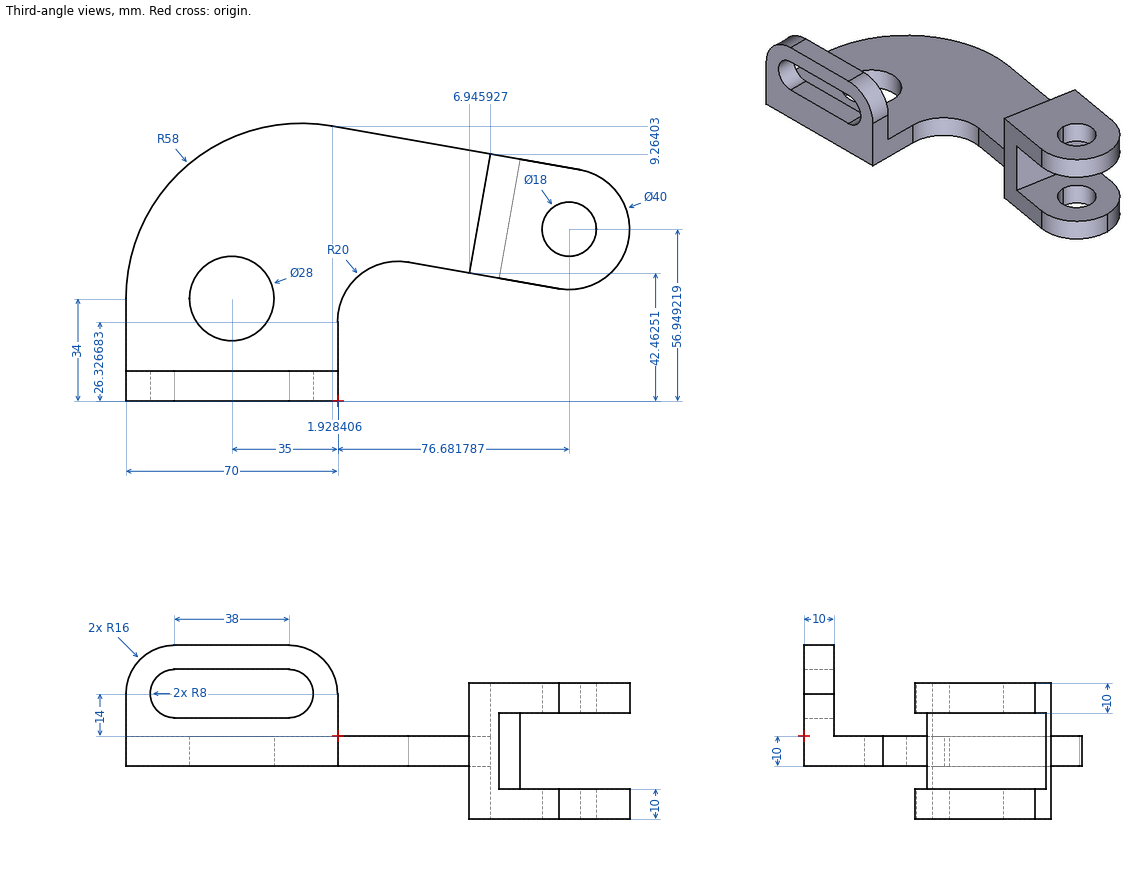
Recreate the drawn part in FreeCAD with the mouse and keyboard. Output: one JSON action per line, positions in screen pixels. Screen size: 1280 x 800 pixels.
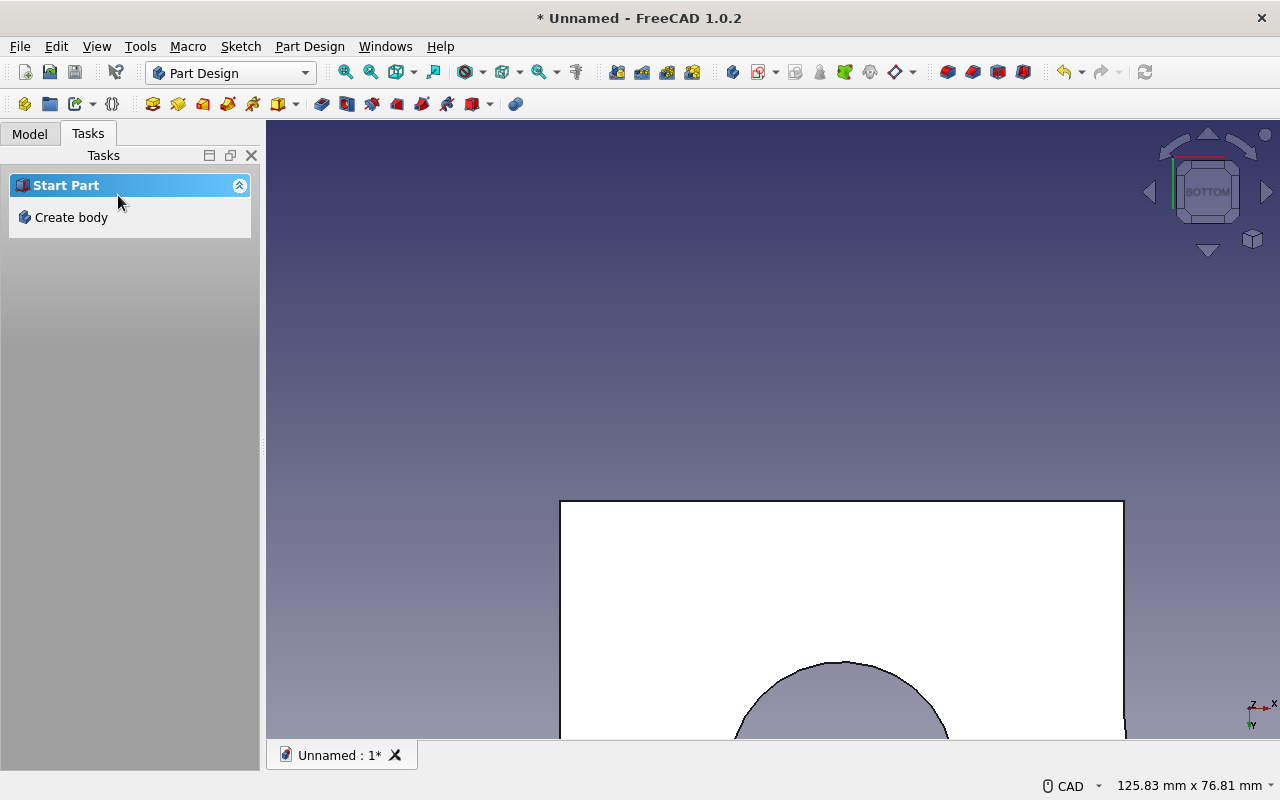
{"action": "left_click", "coordinate": [346, 72]}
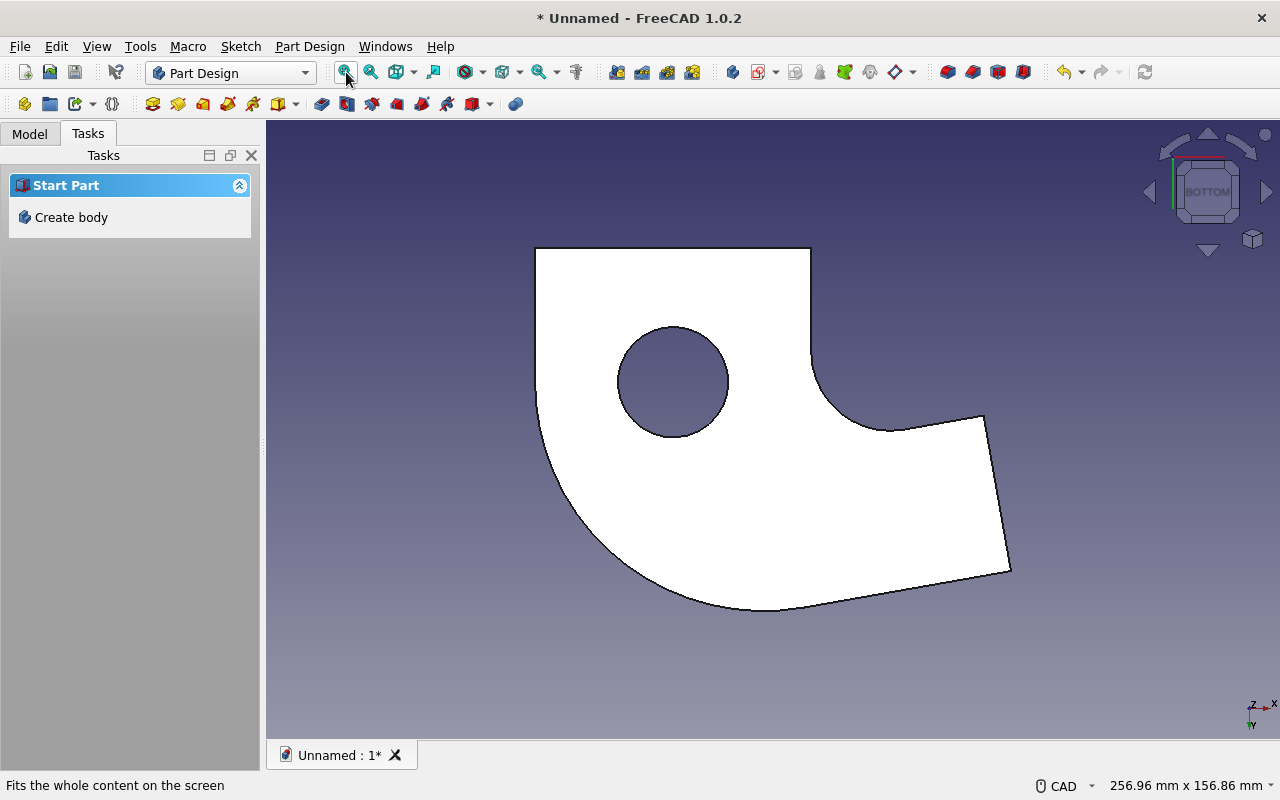
{"action": "key", "text": "4"}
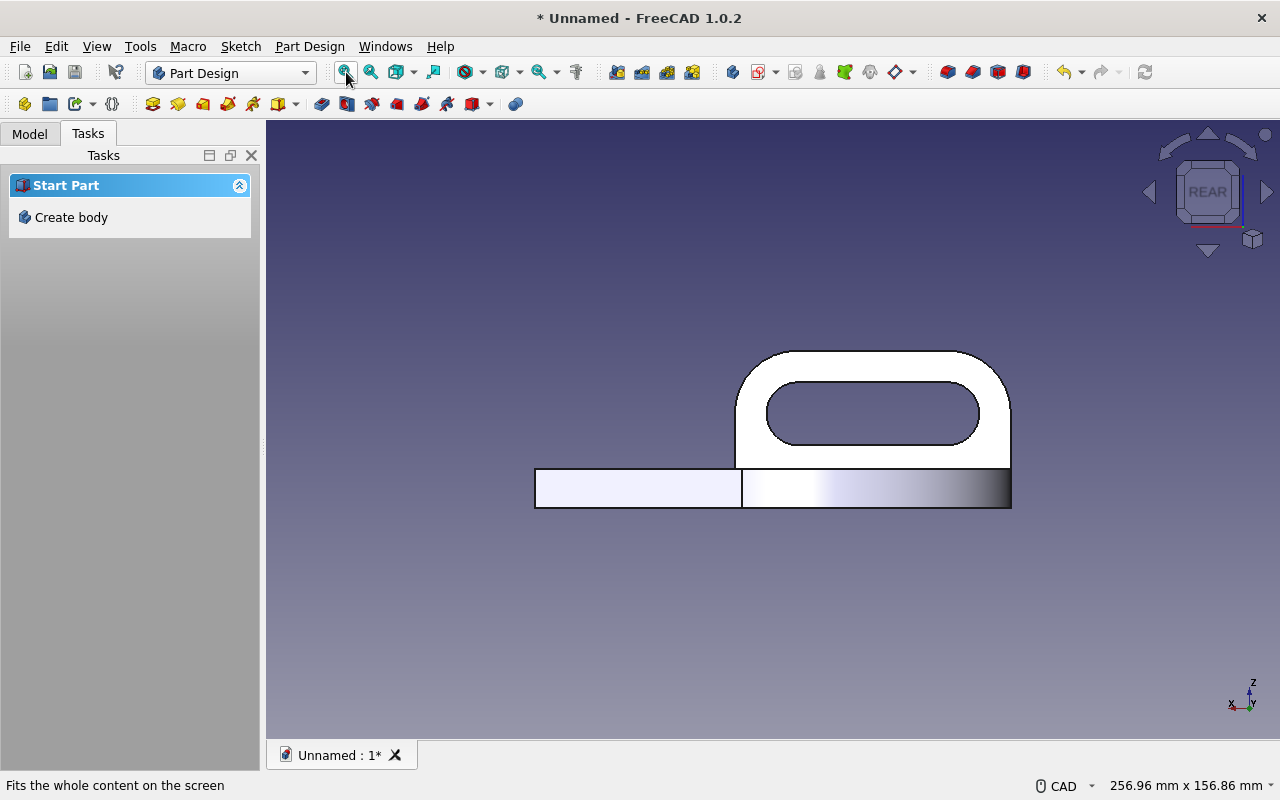
{"action": "left_click", "coordinate": [579, 488]}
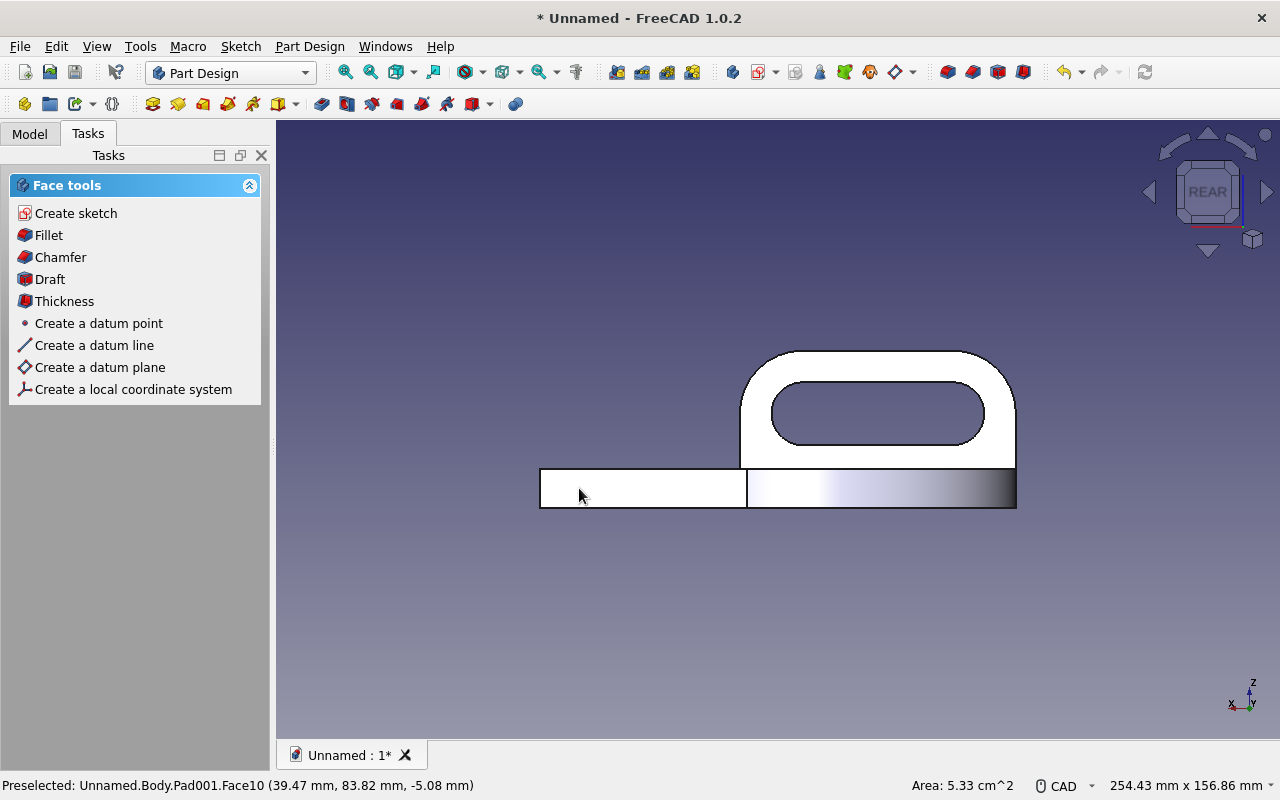
{"action": "left_click", "coordinate": [758, 72]}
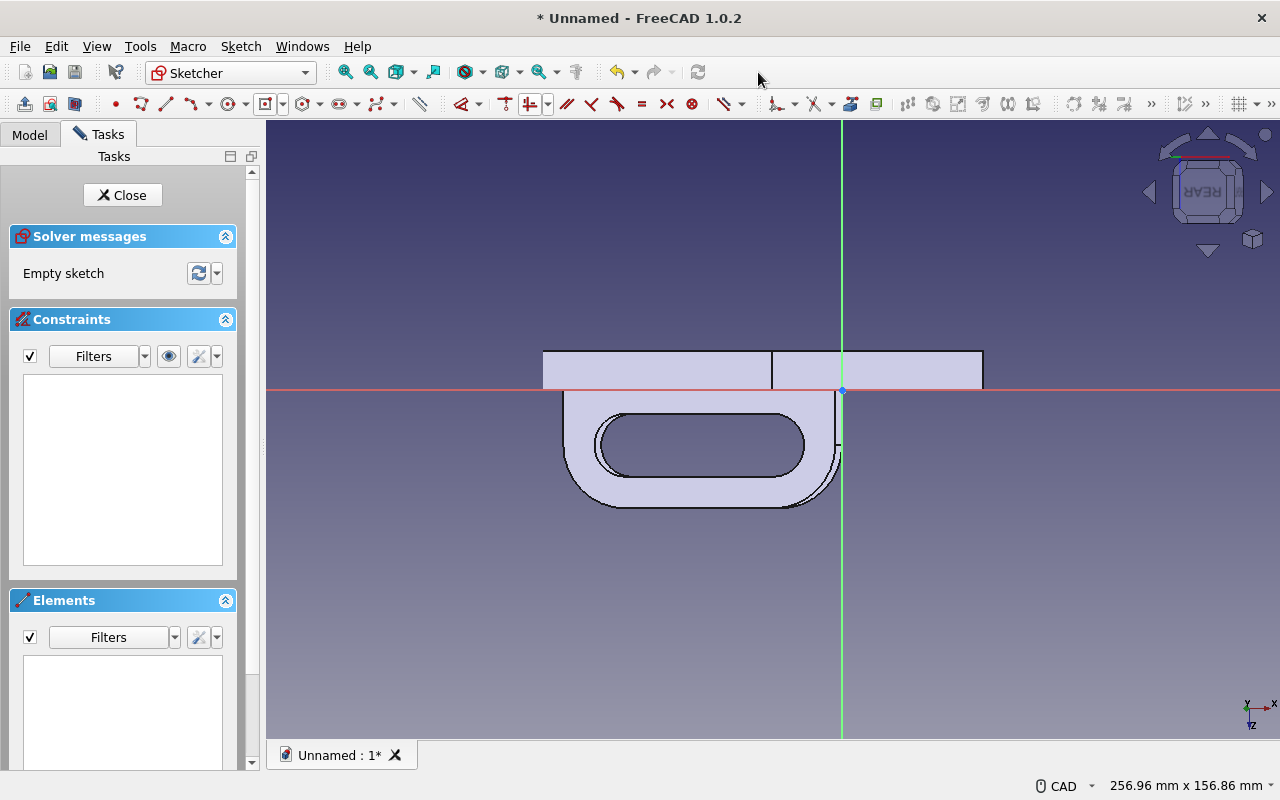
{"action": "left_click", "coordinate": [75, 104]}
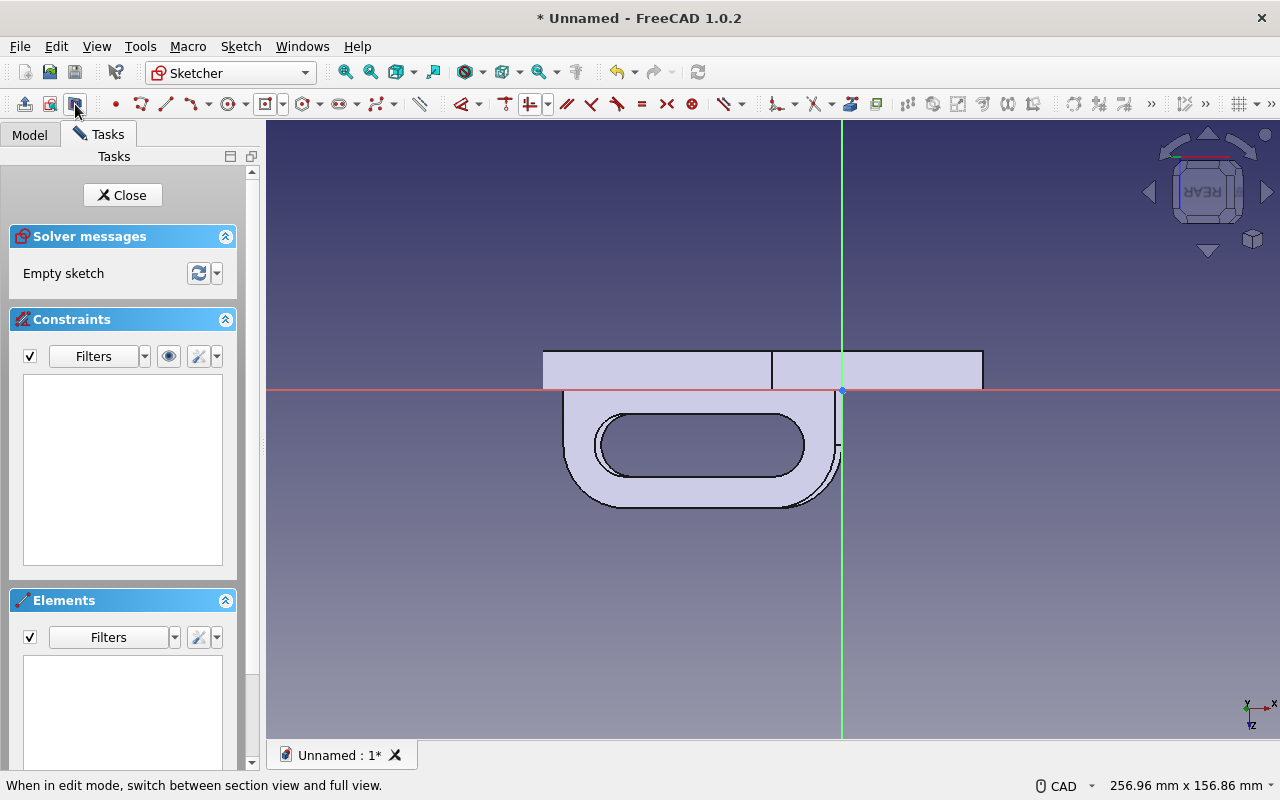
{"action": "scroll", "coordinate": [1115, 322], "scroll_direction": "up", "scroll_amount": 4}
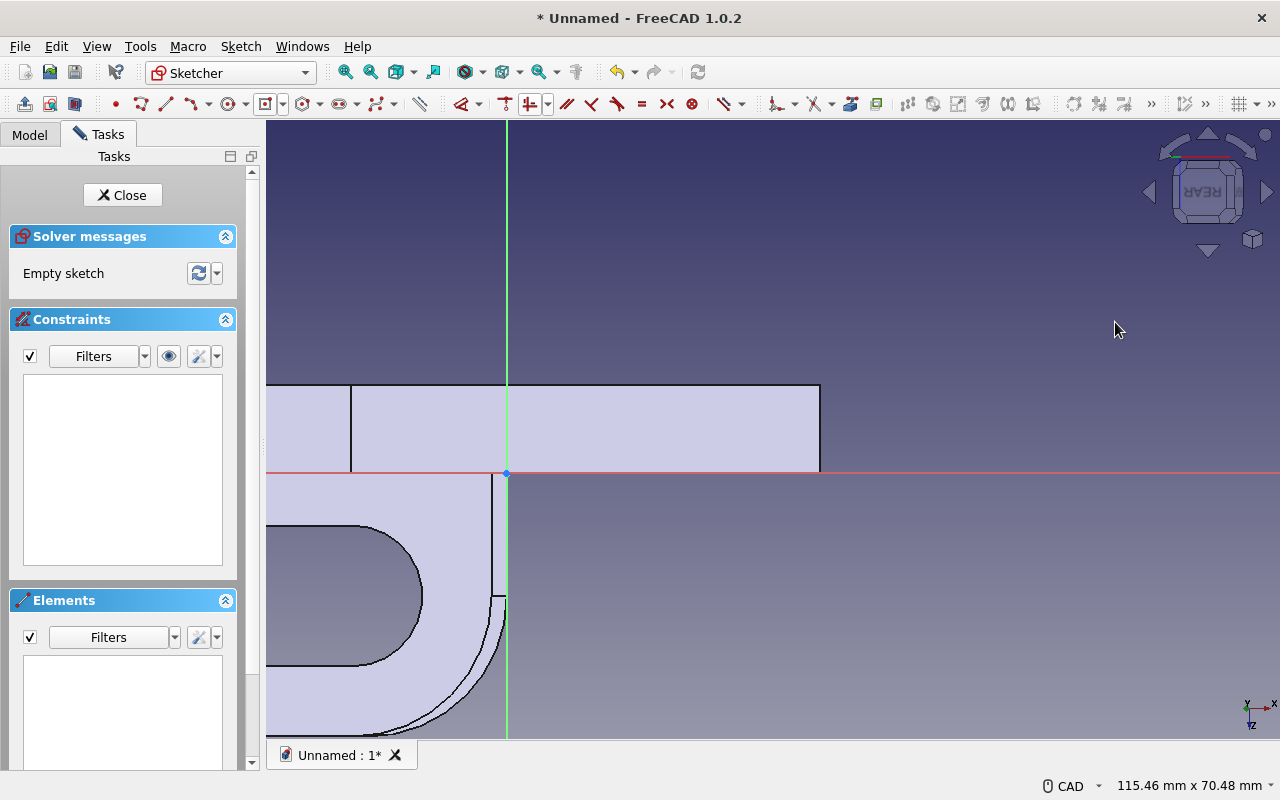
{"action": "left_click", "coordinate": [141, 104]}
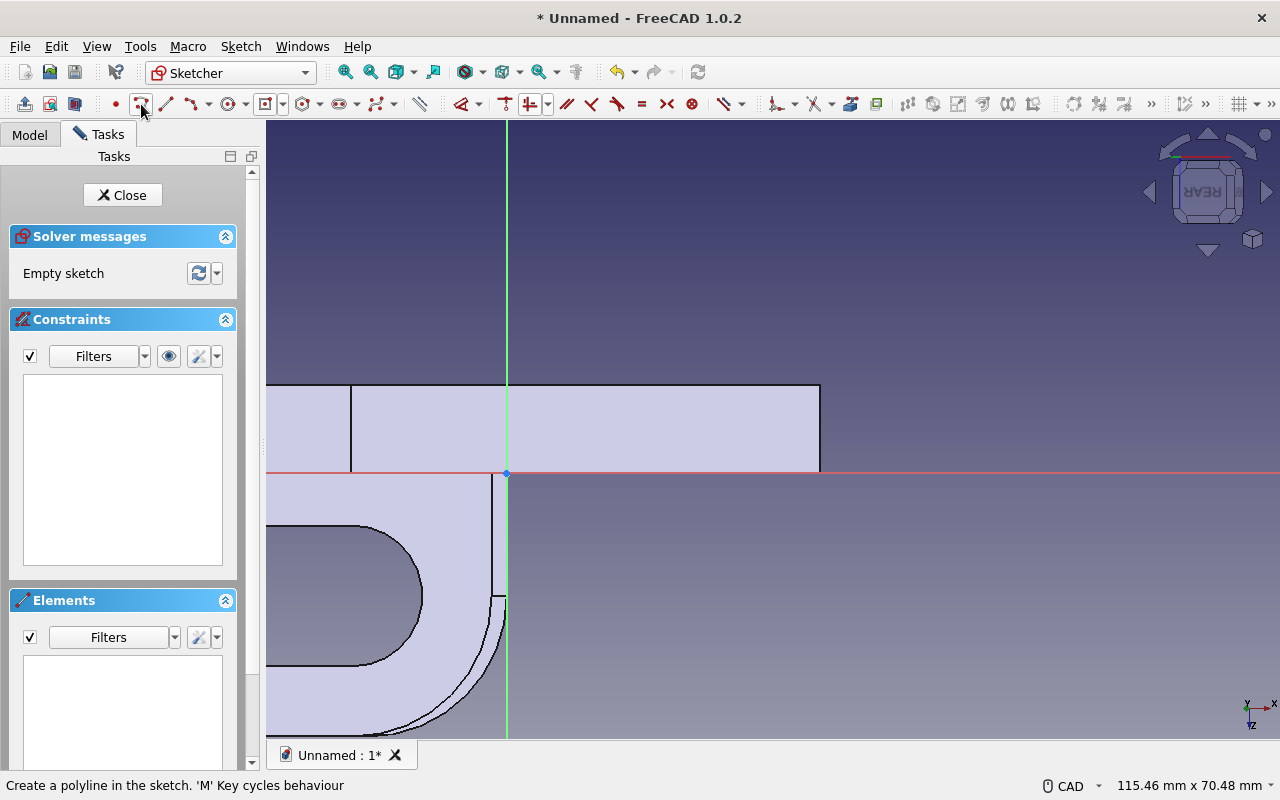
{"action": "left_click", "coordinate": [820, 627]}
{"action": "left_click", "coordinate": [1083, 627]}
{"action": "left_click", "coordinate": [1083, 539]}
{"action": "left_click", "coordinate": [908, 539]}
{"action": "left_click", "coordinate": [908, 319]}
{"action": "left_click", "coordinate": [1083, 319]}
{"action": "left_click", "coordinate": [1083, 232]}
{"action": "left_click", "coordinate": [820, 232]}
{"action": "left_click", "coordinate": [820, 628]}
{"action": "key", "text": "Escape"}
{"action": "key", "text": "Escape"}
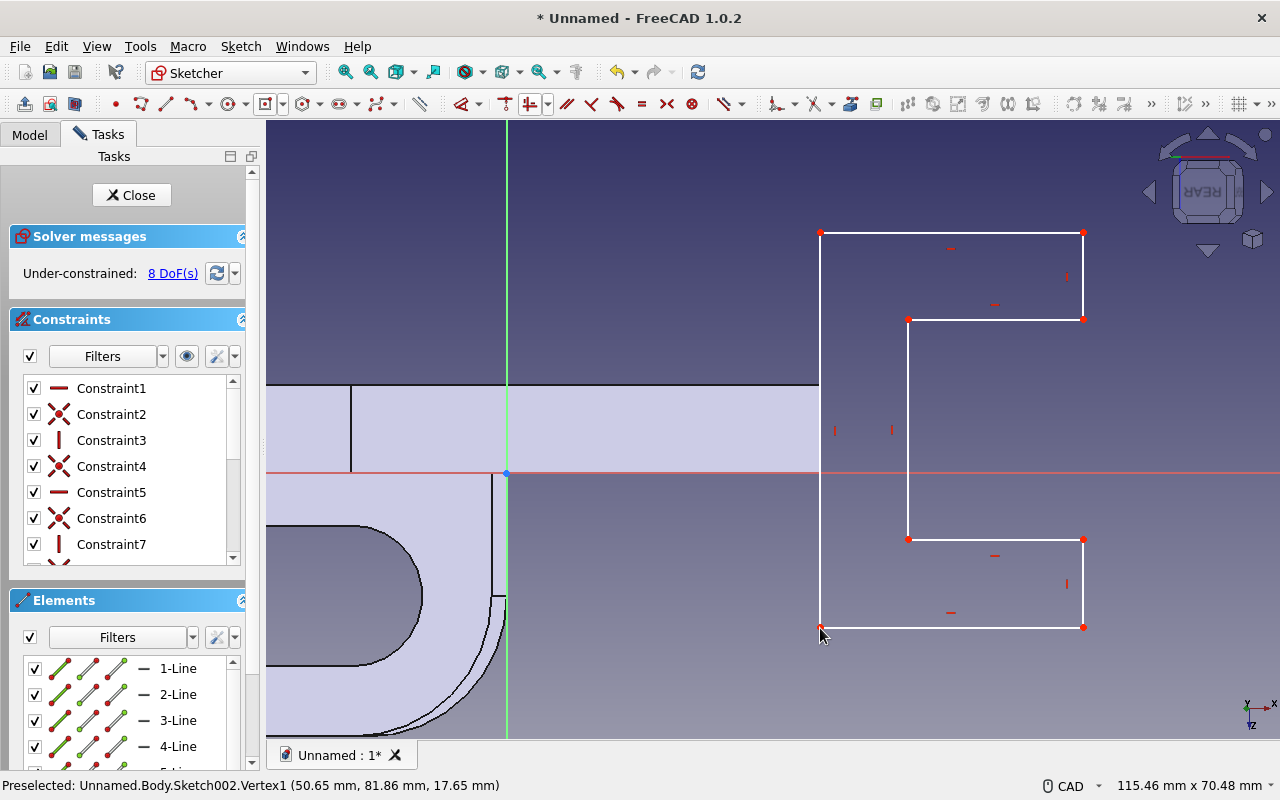
{"action": "left_click", "coordinate": [1083, 628]}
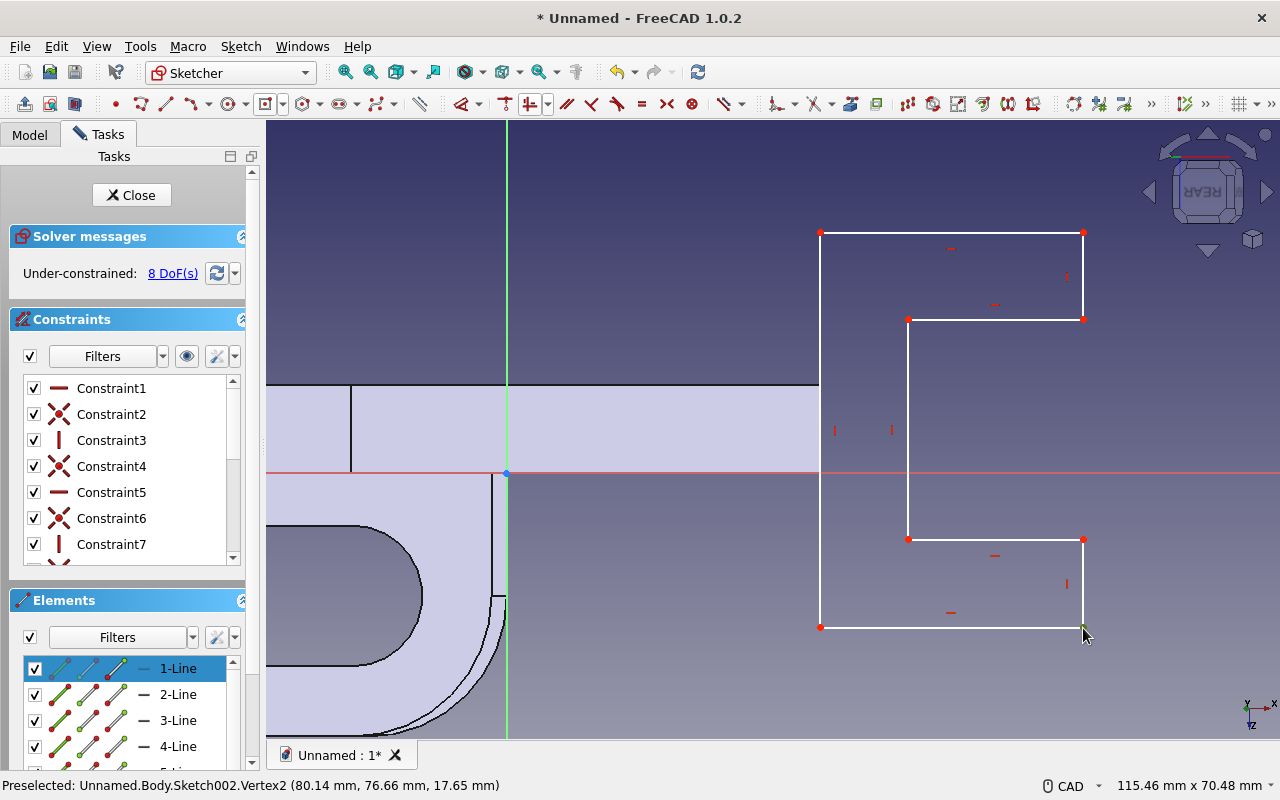
{"action": "left_click", "coordinate": [1083, 320]}